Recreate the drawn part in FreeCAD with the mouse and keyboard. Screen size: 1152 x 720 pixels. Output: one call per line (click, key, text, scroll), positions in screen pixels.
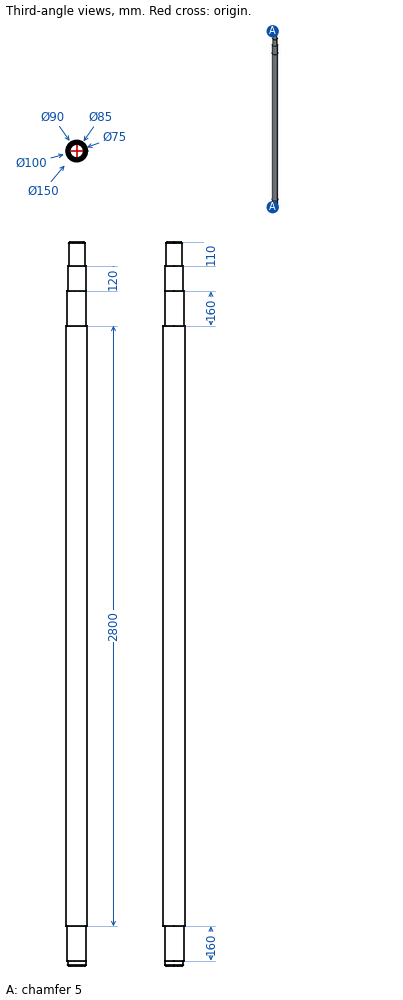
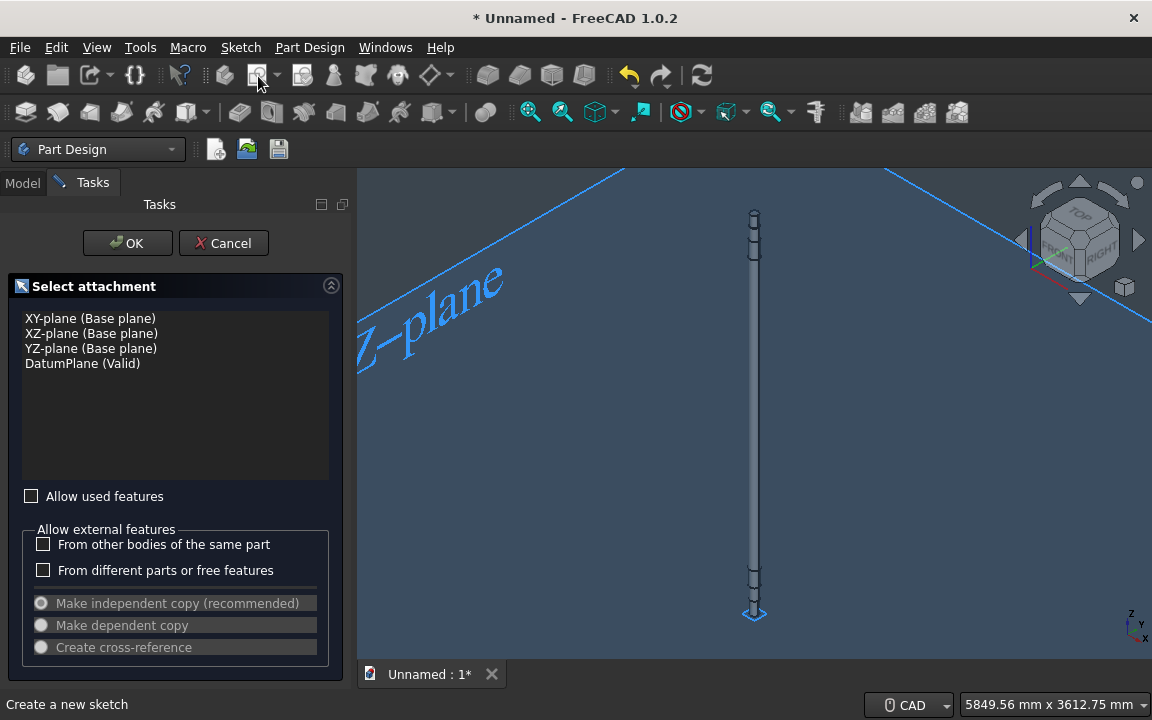
click(82, 318)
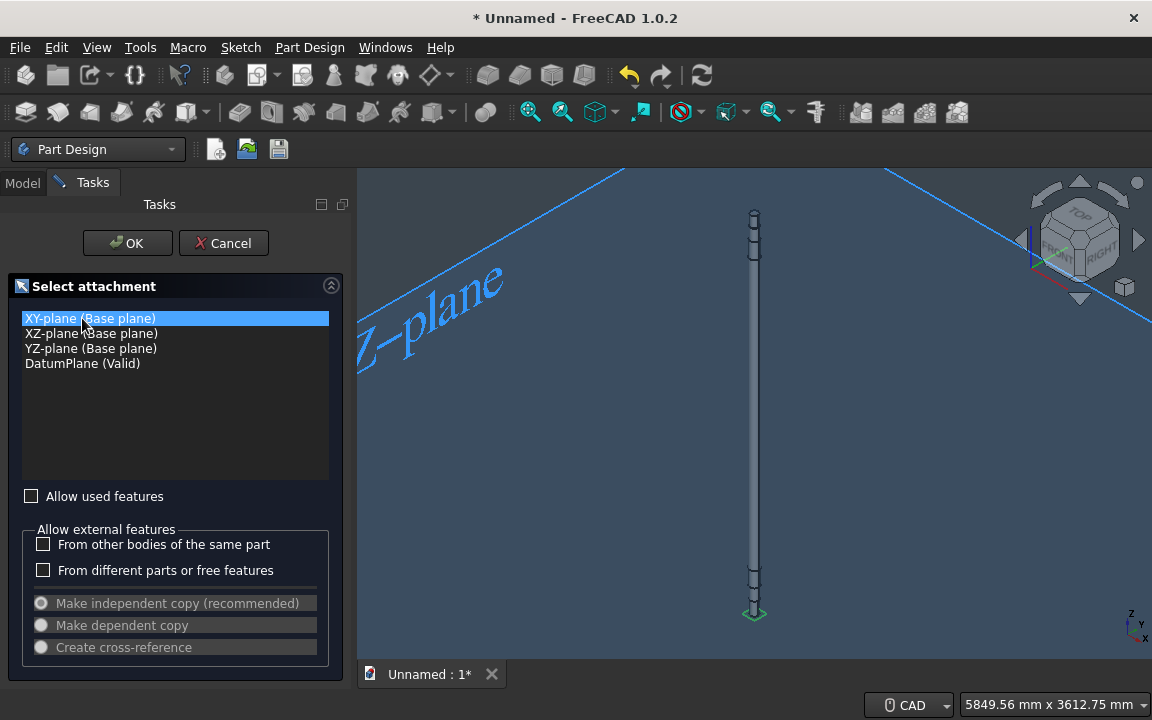
click(128, 243)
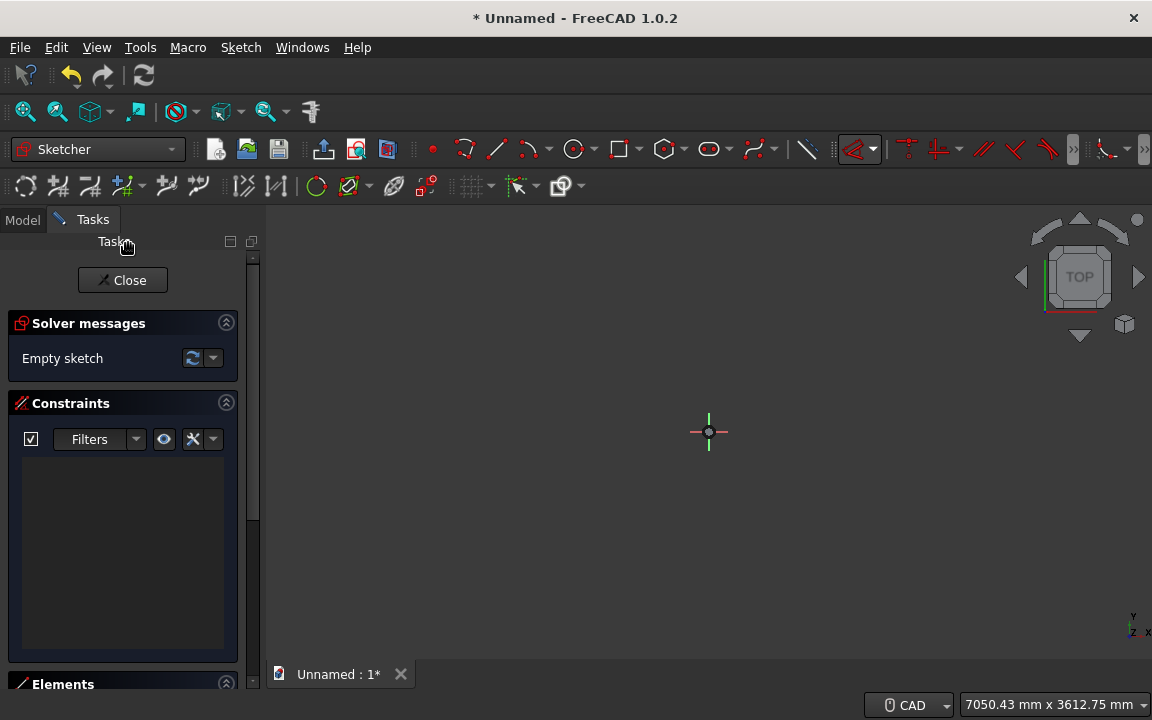
key(q)
key(s)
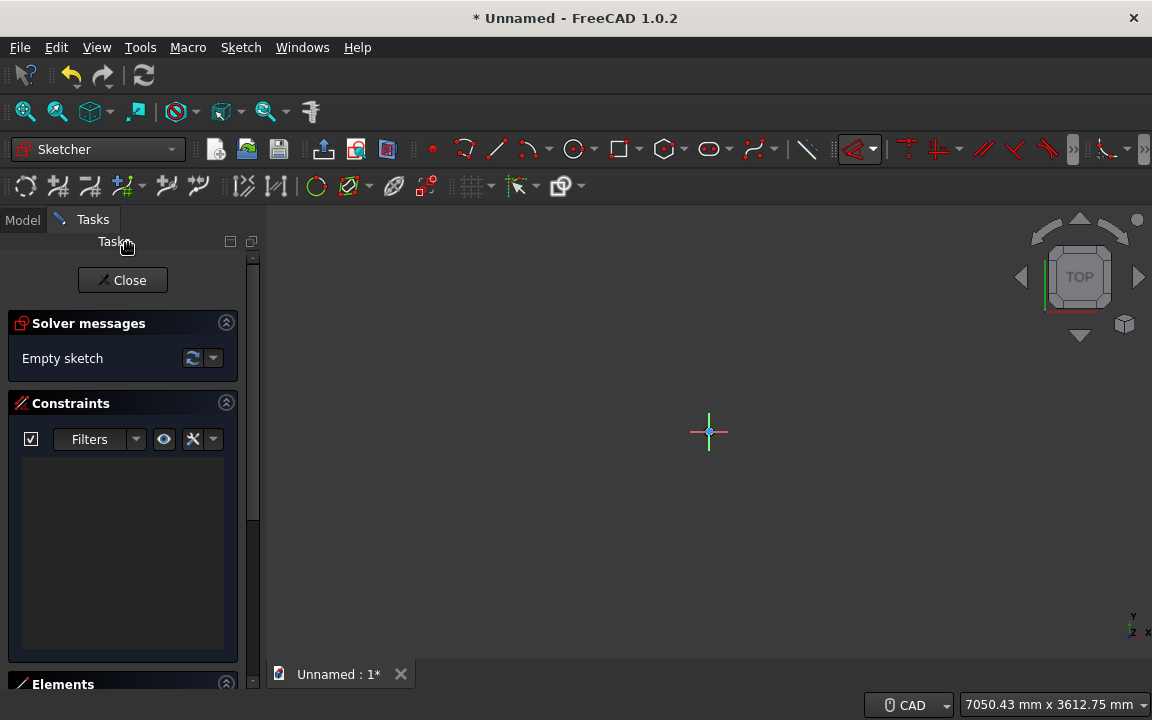
scroll(713, 432, up, 14)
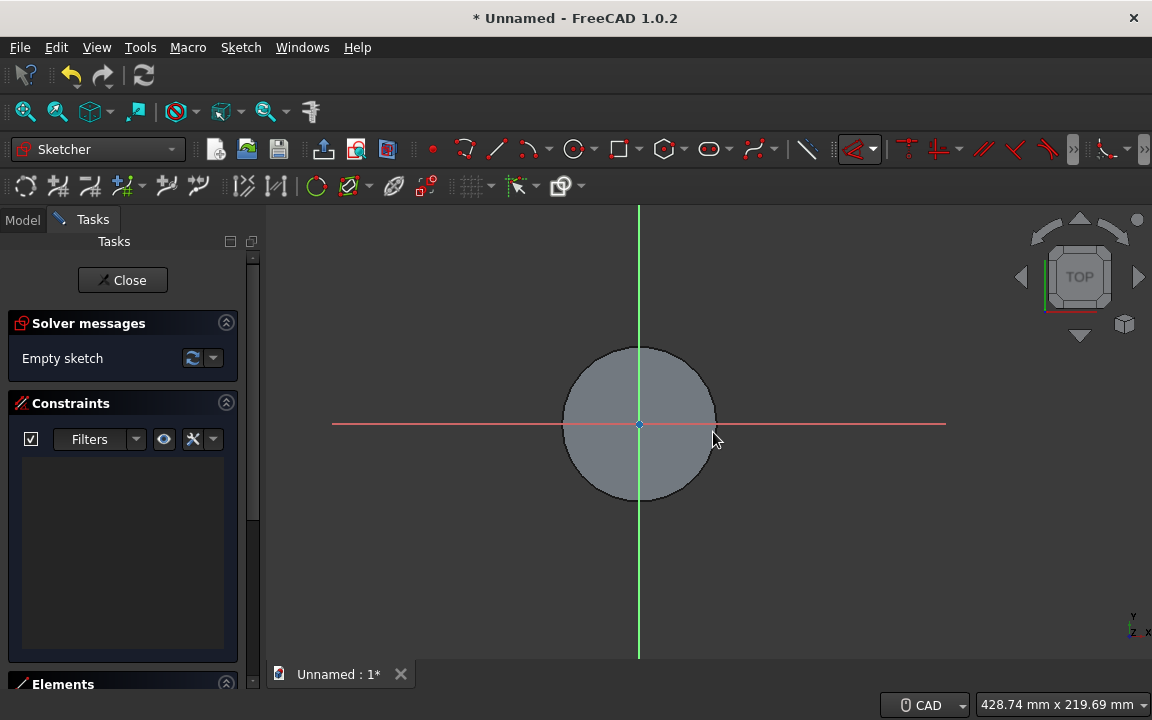
click(574, 150)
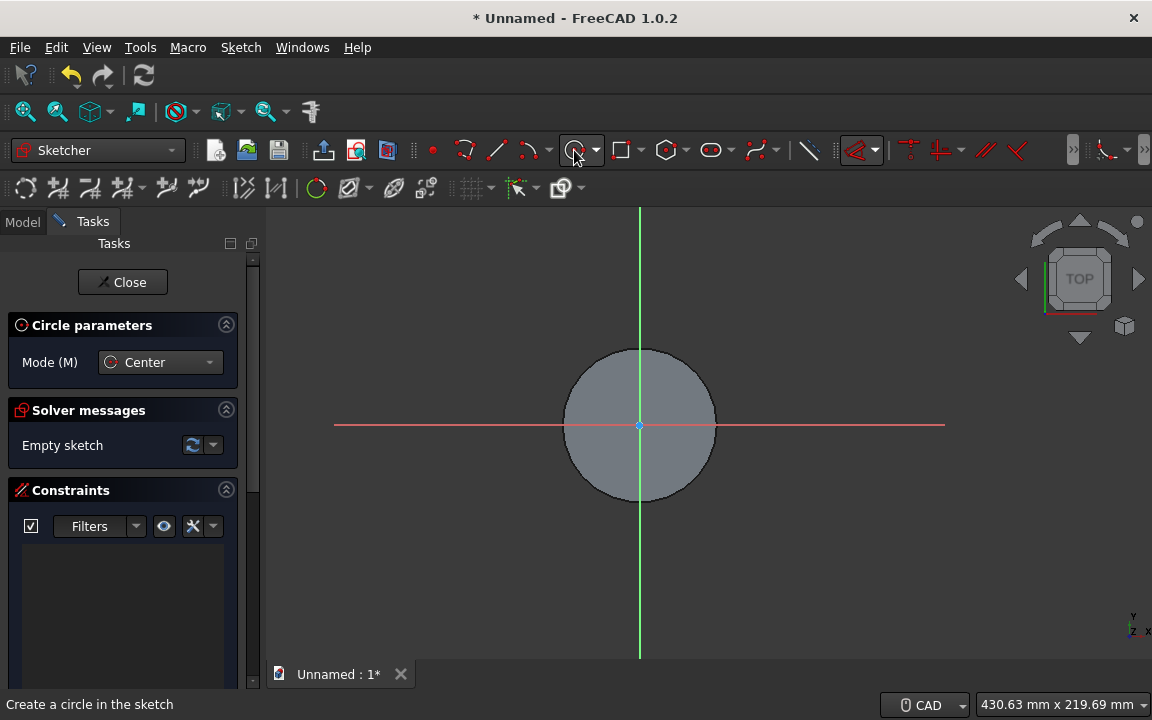
click(640, 425)
click(749, 316)
key(Escape)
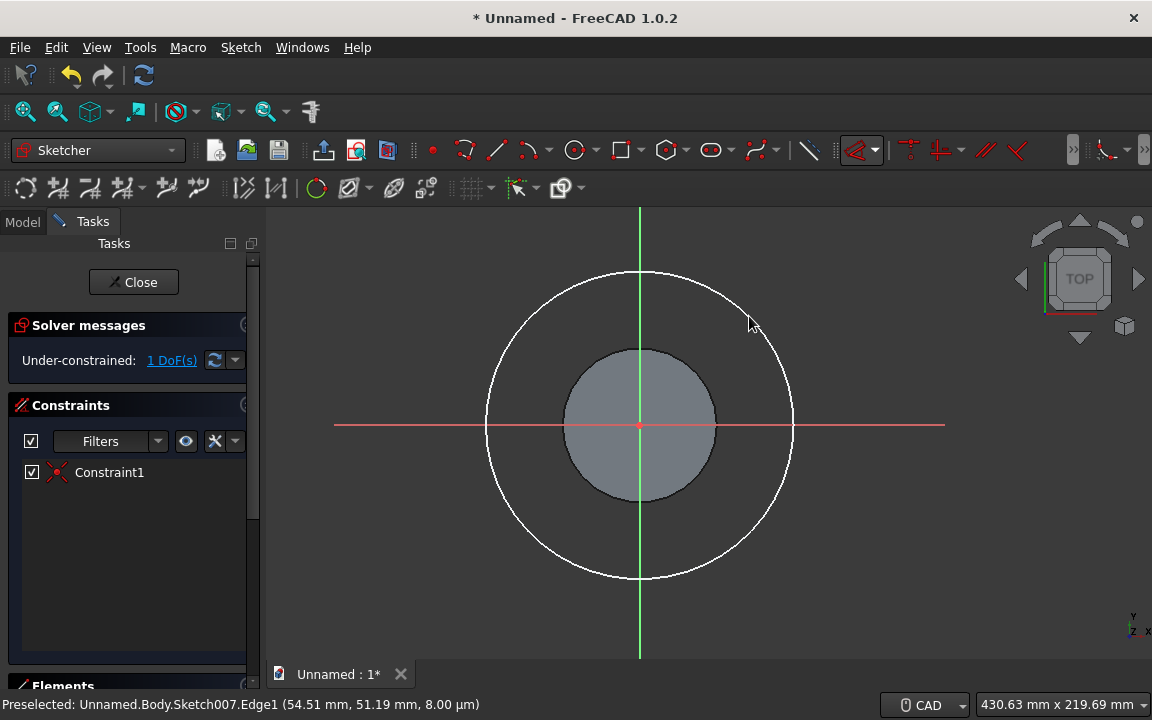
click(748, 316)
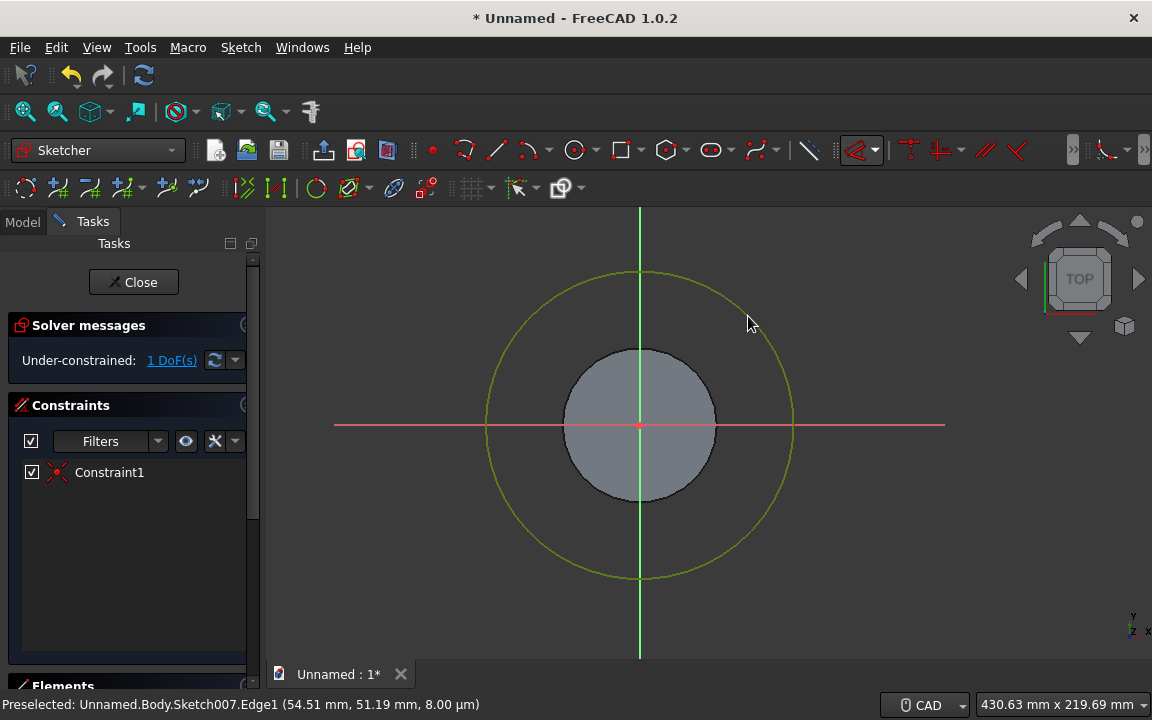
key(k)
key(o)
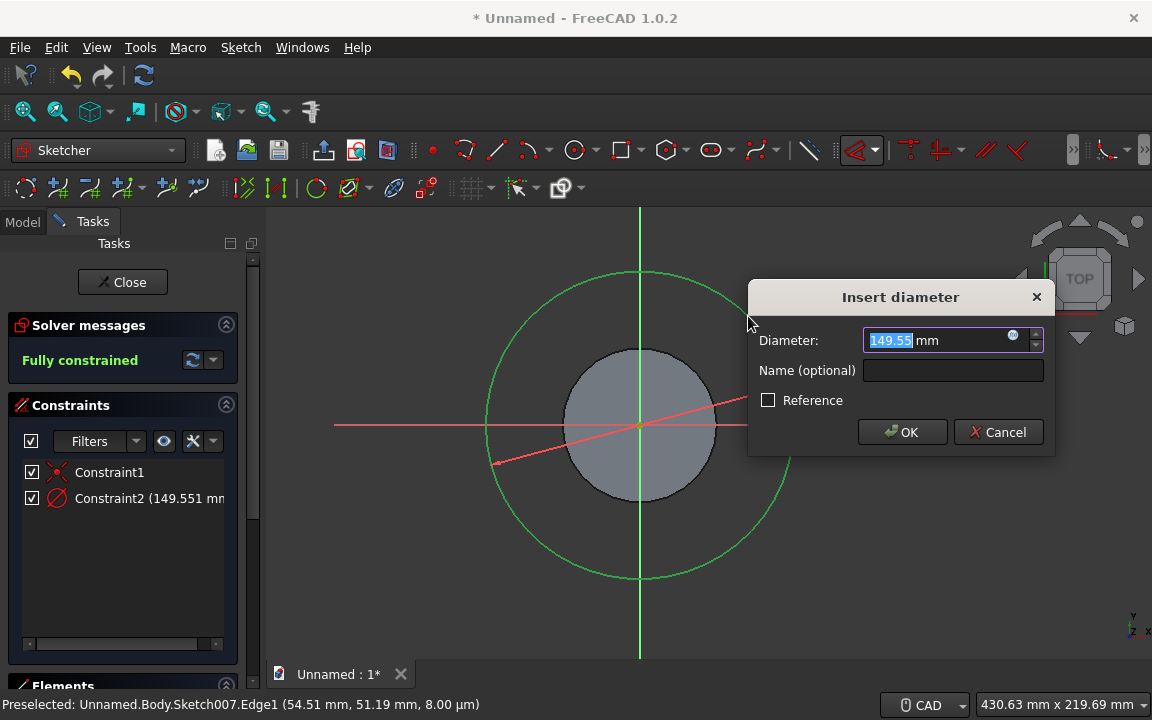
text(150)
key(Return)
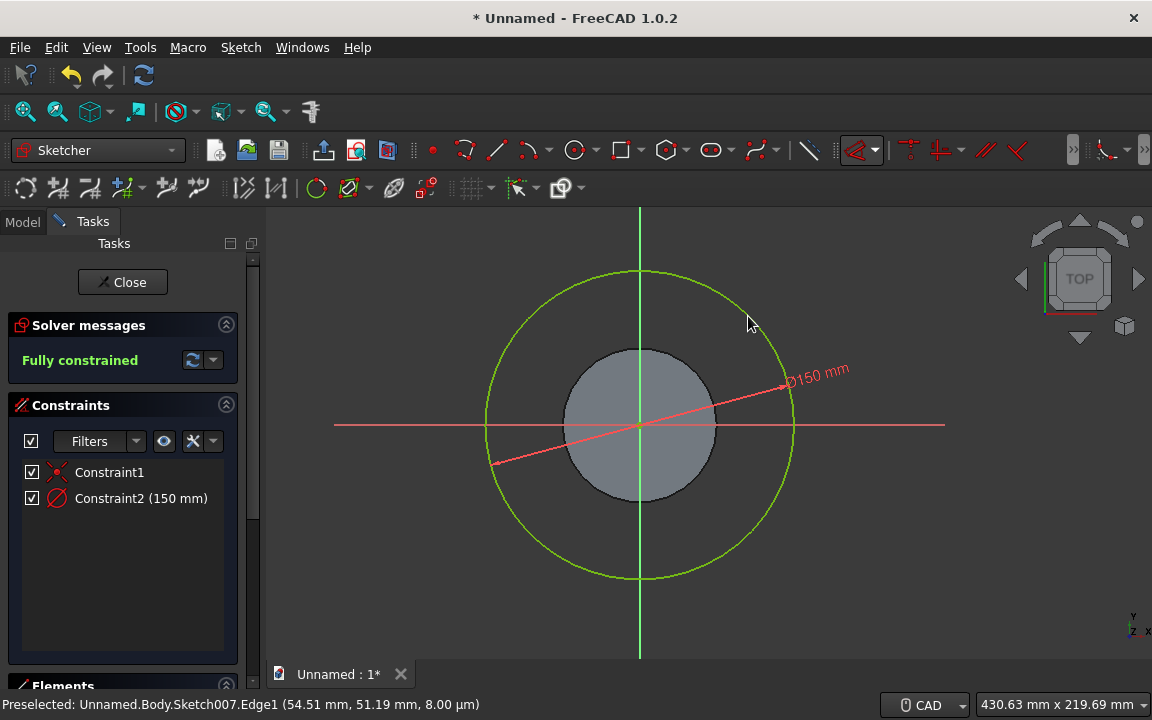
click(123, 282)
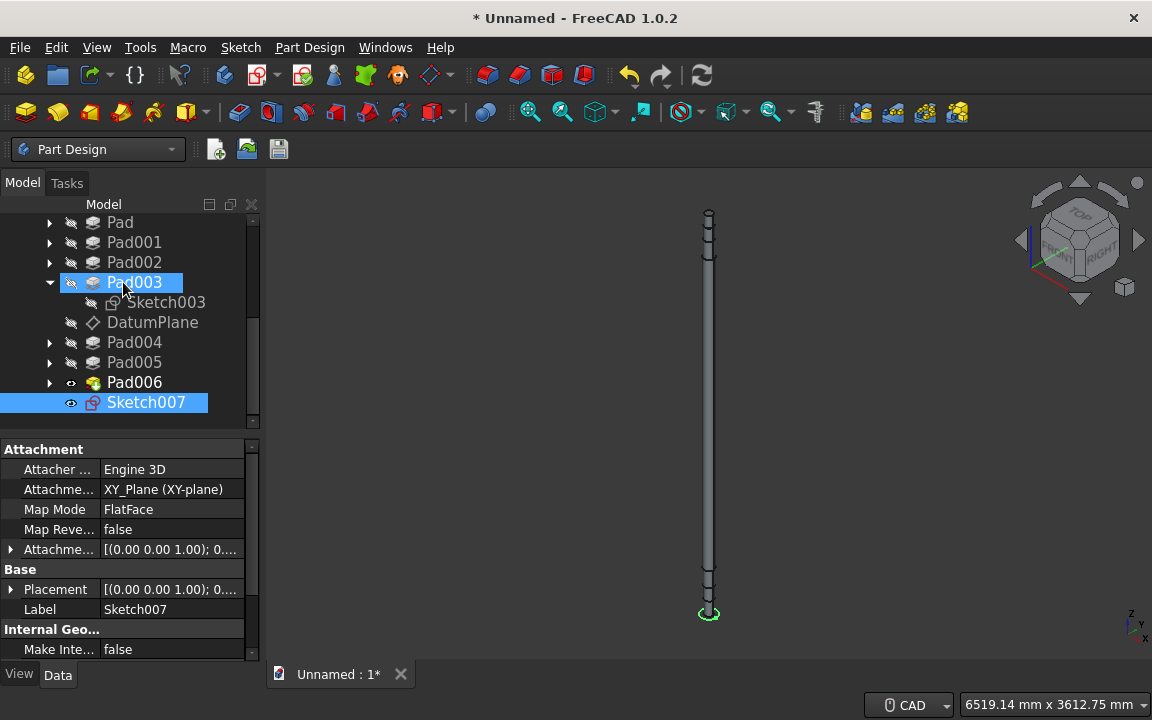
click(240, 112)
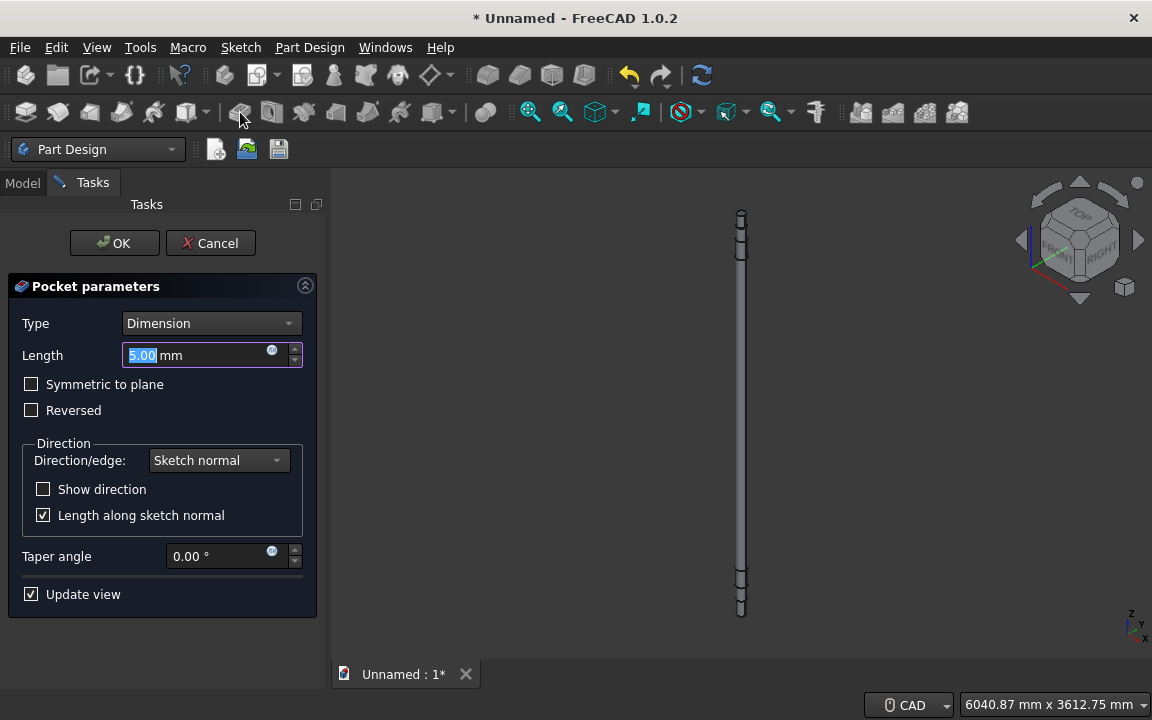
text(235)
key(Tab)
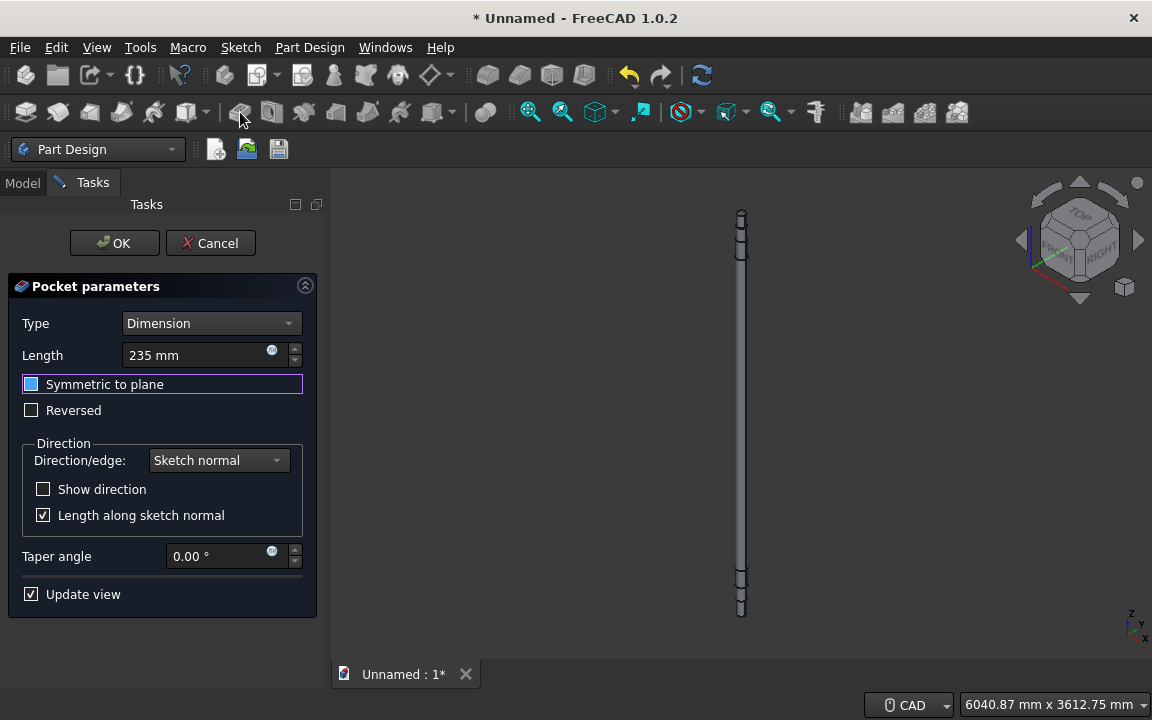
click(30, 410)